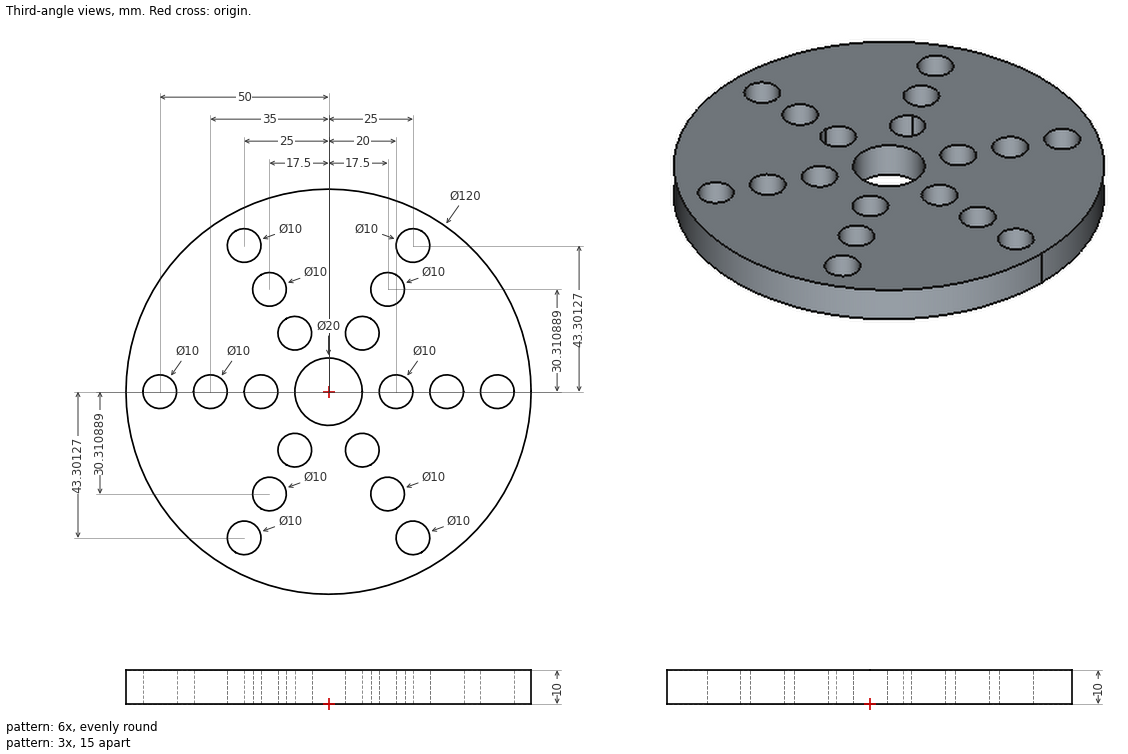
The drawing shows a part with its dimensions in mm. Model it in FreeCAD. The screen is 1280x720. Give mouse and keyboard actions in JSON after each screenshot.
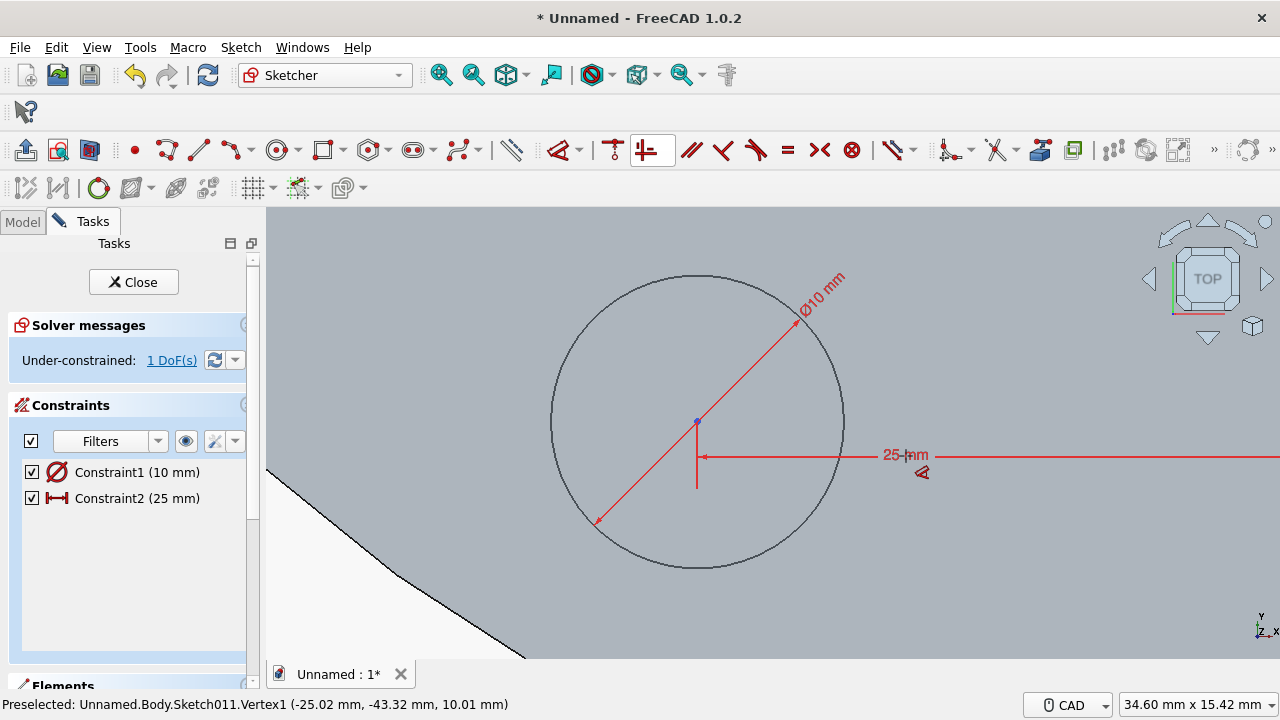
{"action": "left_click", "coordinate": [697, 422]}
{"action": "left_click", "coordinate": [663, 328]}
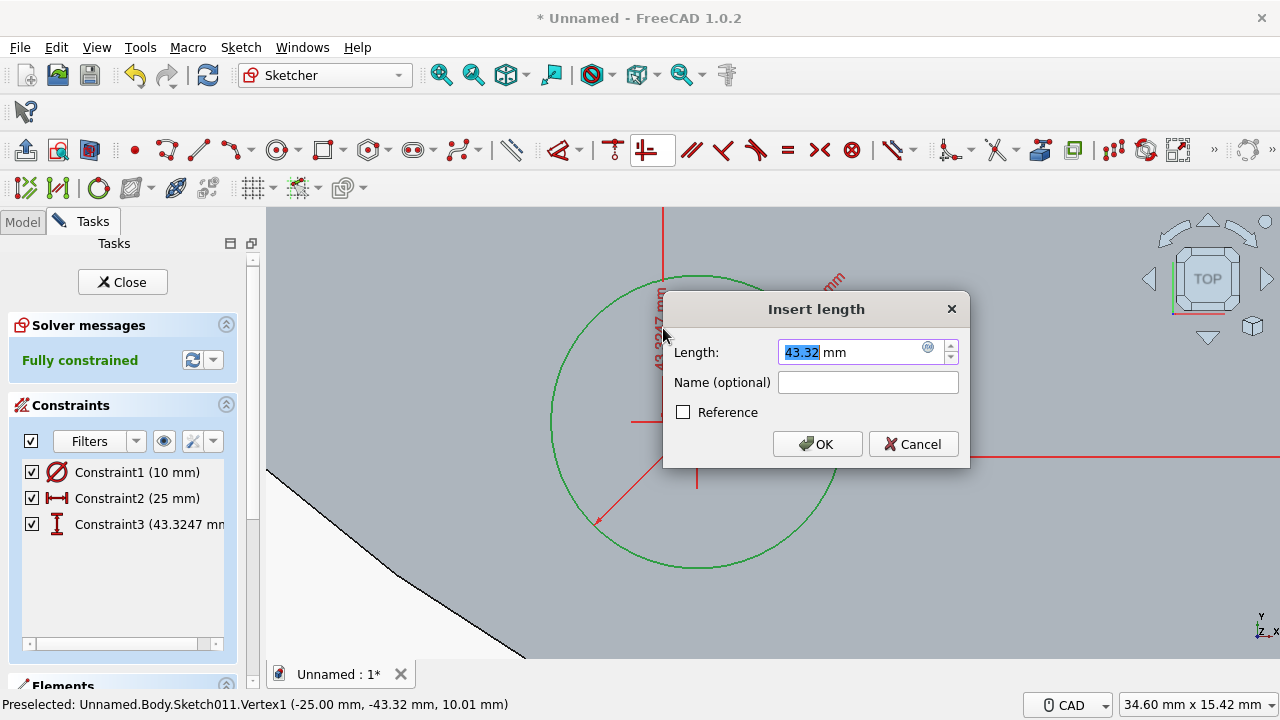
{"action": "type", "text": "43.30127"}
{"action": "key", "text": "Return"}
{"action": "key", "text": "Escape"}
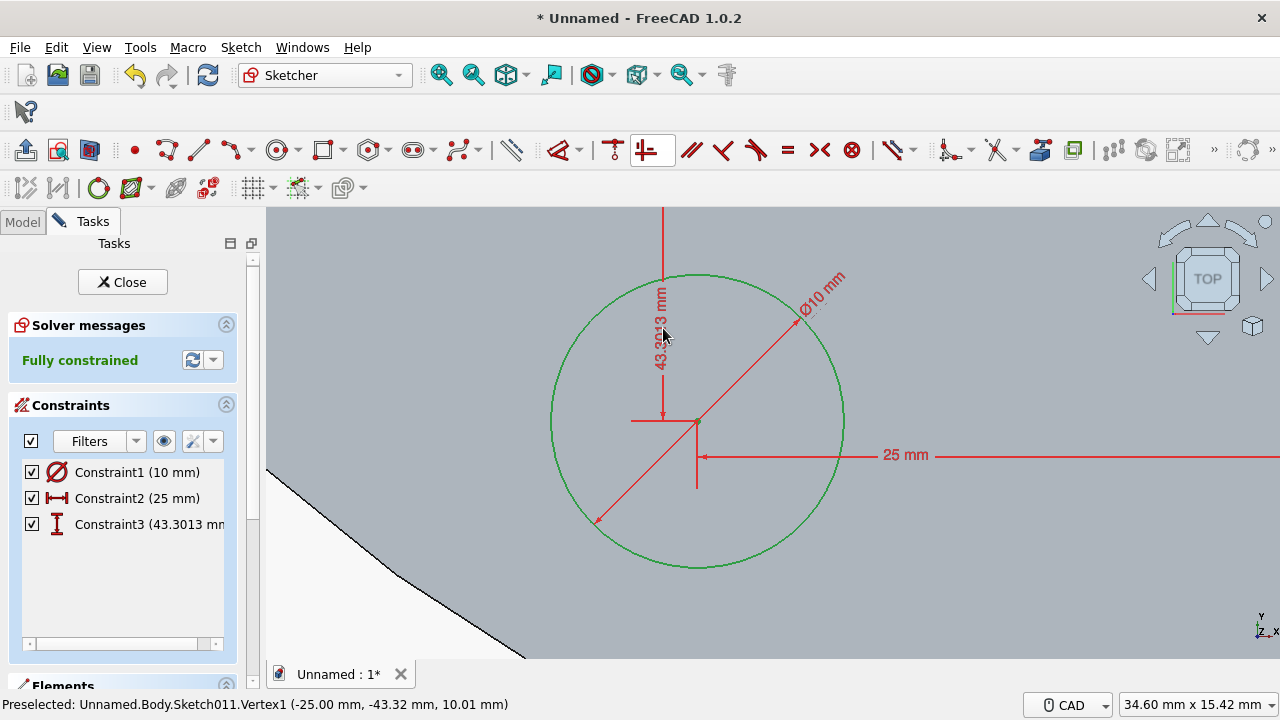
{"action": "left_click", "coordinate": [123, 282]}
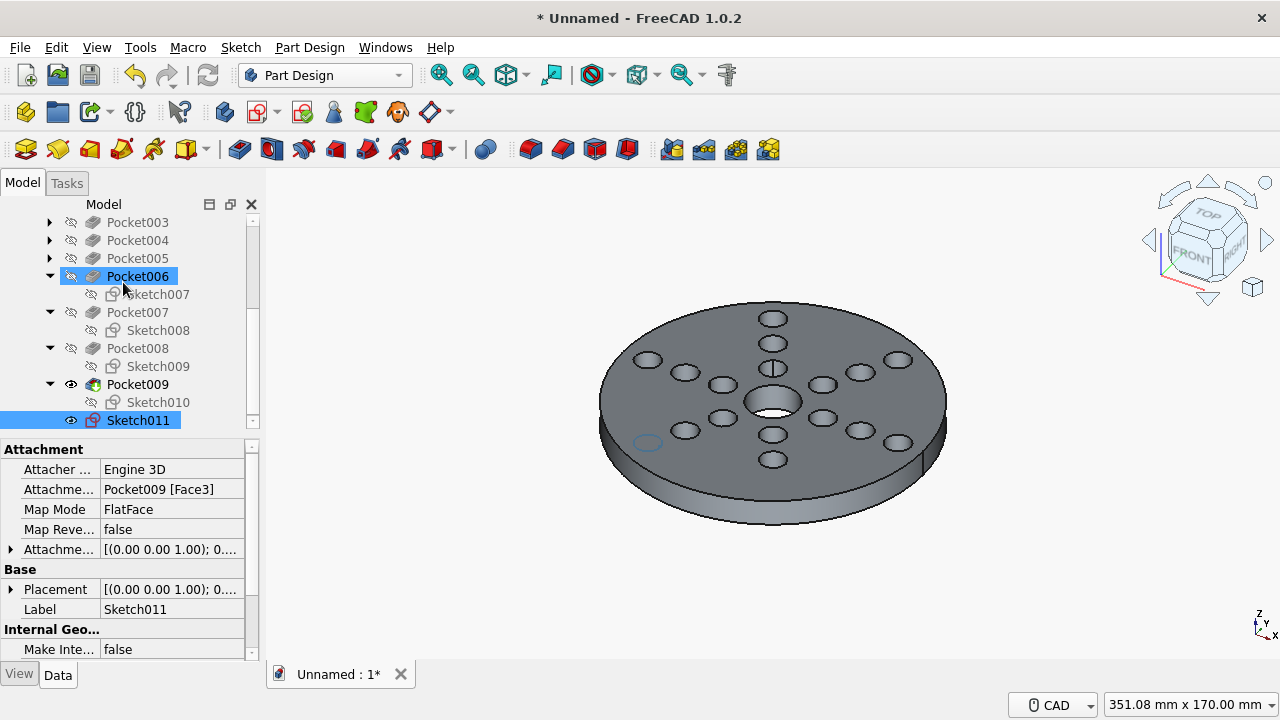
{"action": "left_click", "coordinate": [240, 150]}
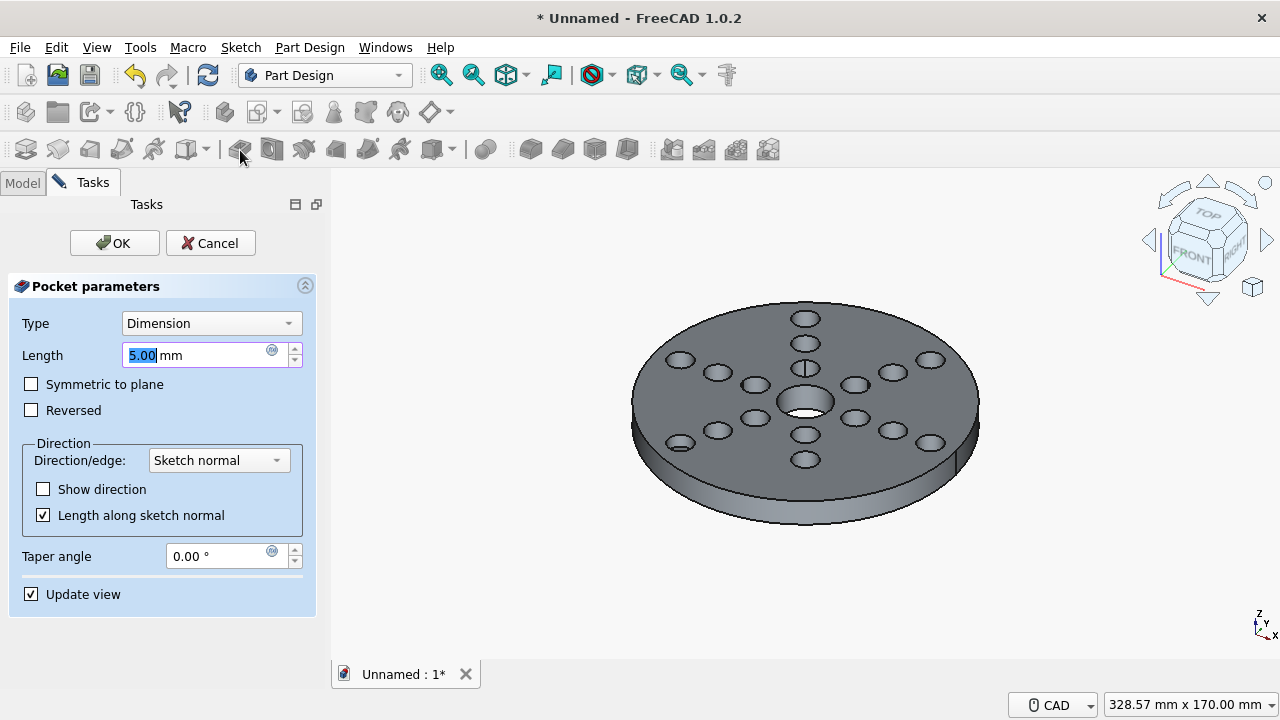
{"action": "type", "text": "10"}
{"action": "key", "text": "Tab"}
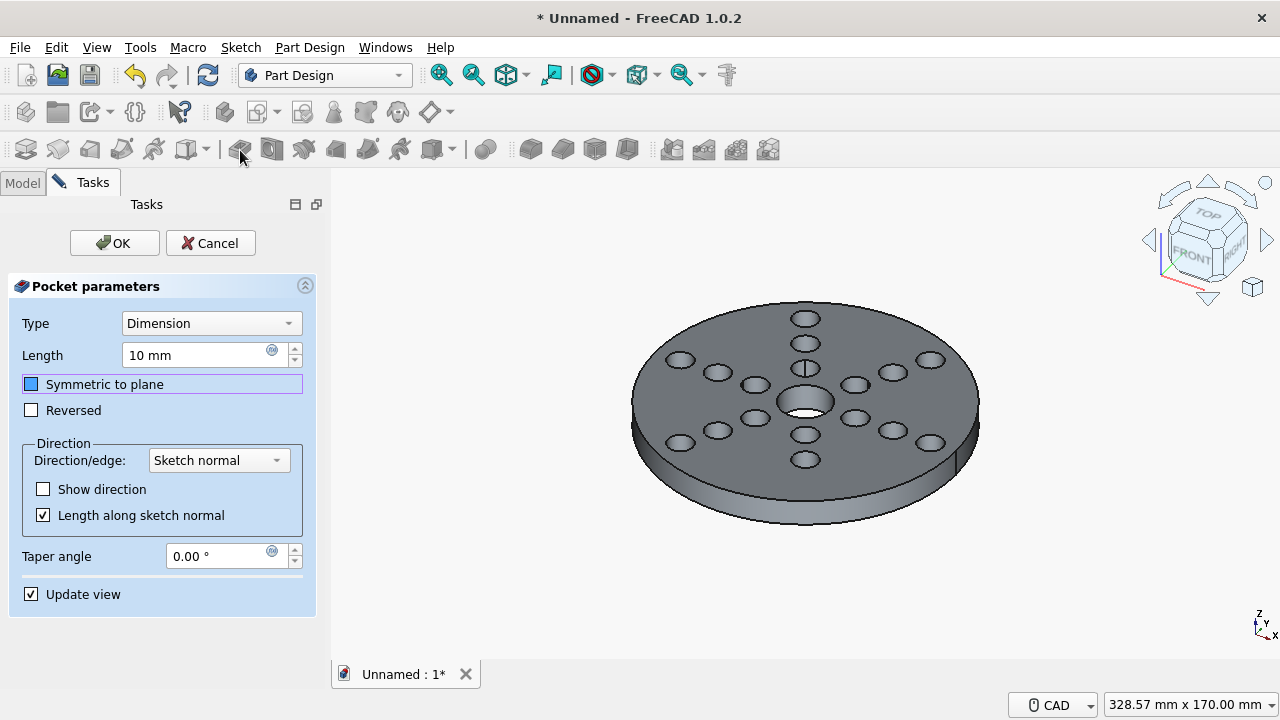
{"action": "left_click", "coordinate": [115, 243]}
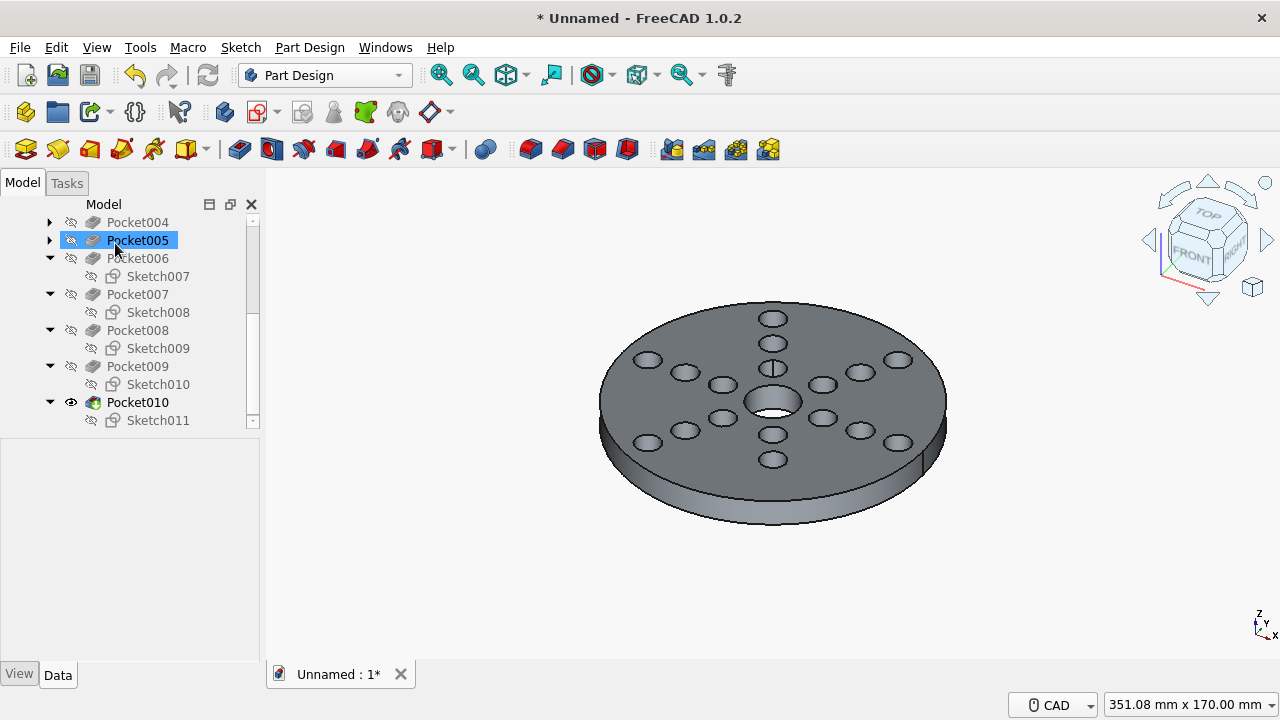
{"action": "left_click", "coordinate": [823, 351]}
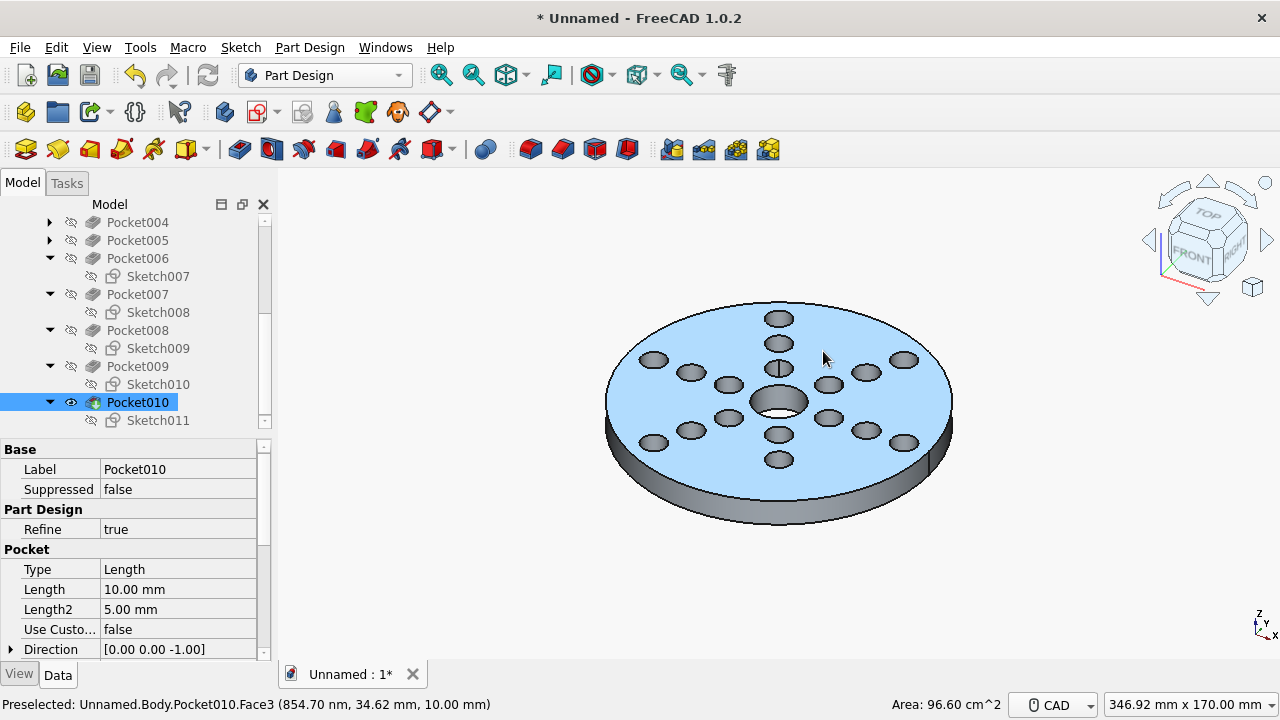
{"action": "left_click", "coordinate": [258, 112]}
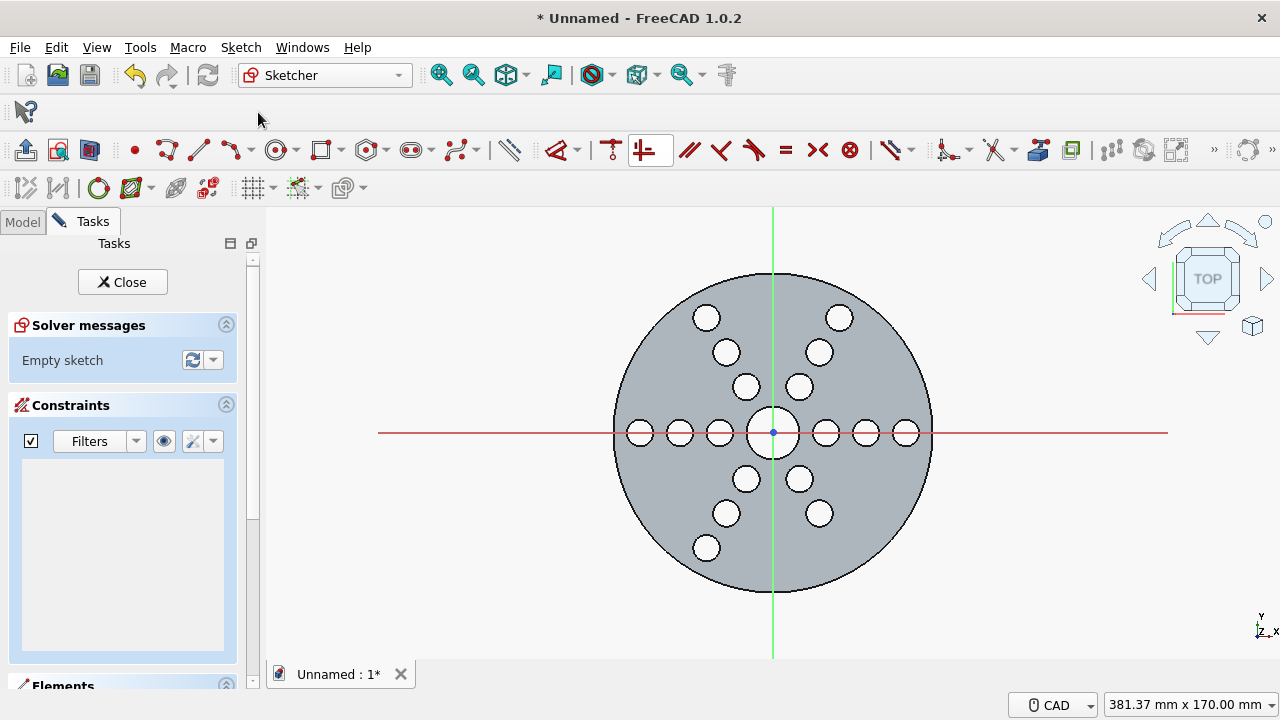
{"action": "scroll", "coordinate": [853, 560], "scroll_direction": "up", "scroll_amount": 12}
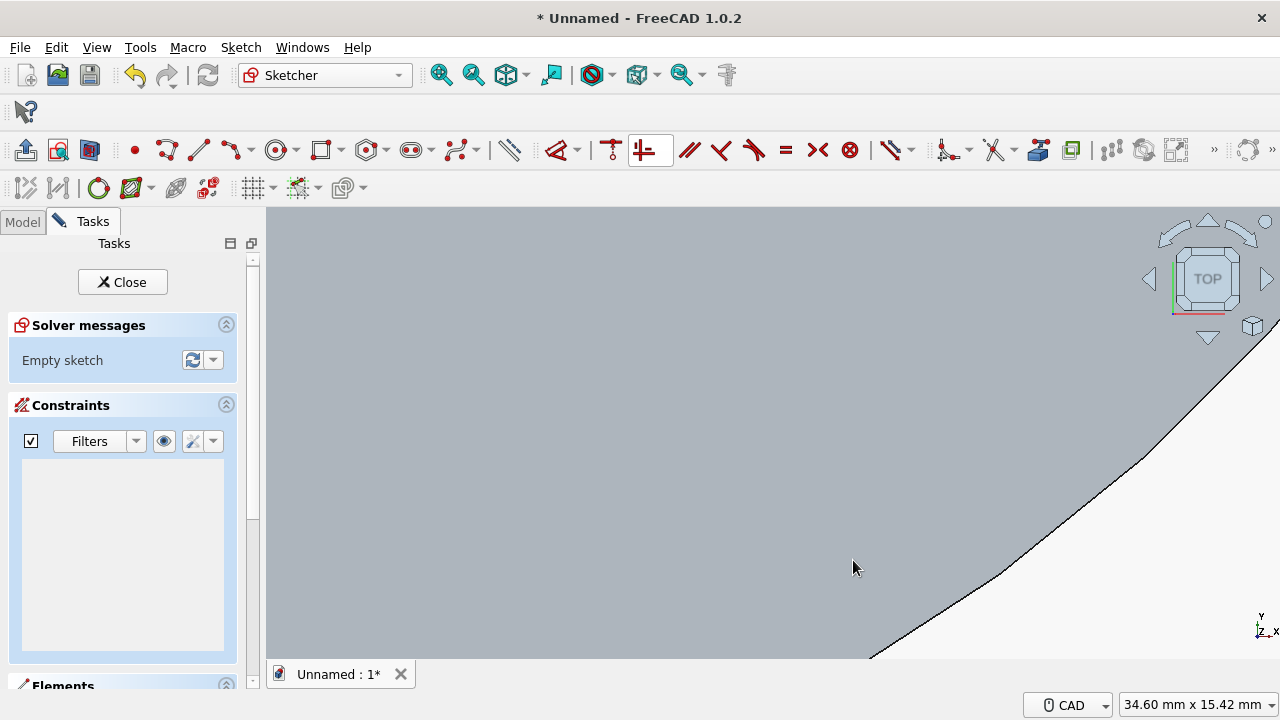
{"action": "left_click", "coordinate": [276, 150]}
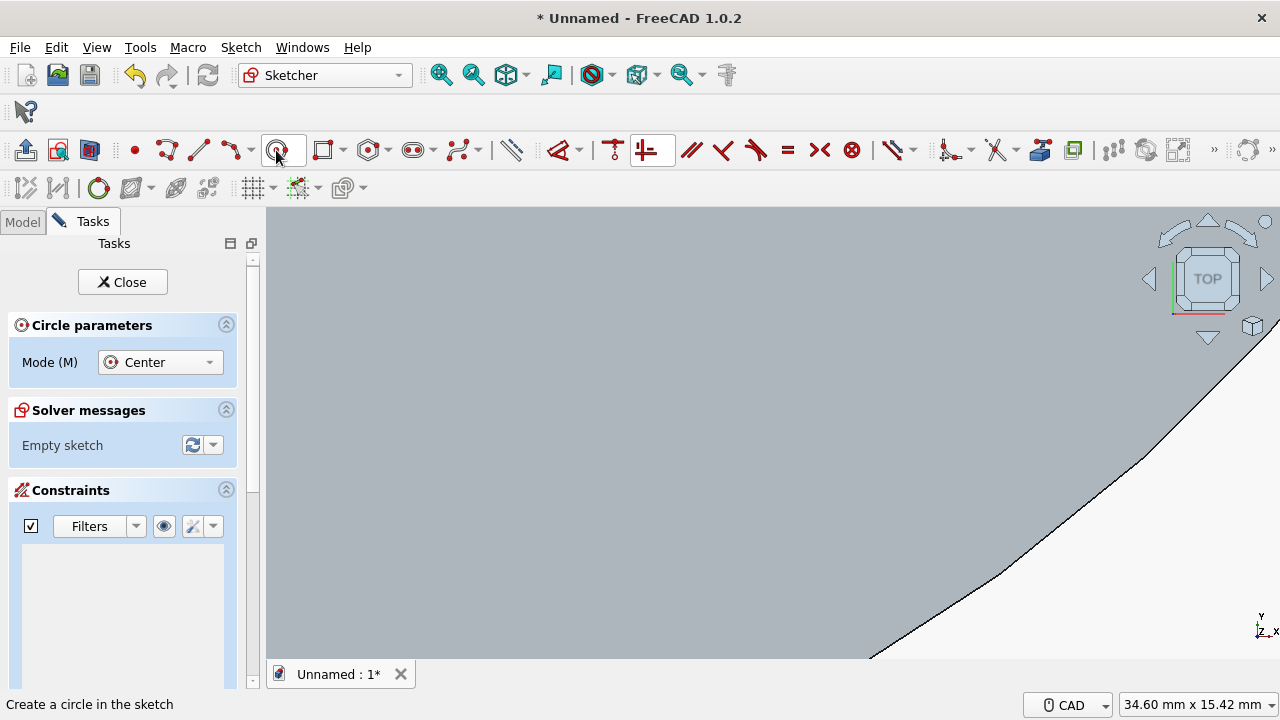
{"action": "left_click", "coordinate": [698, 421]}
{"action": "left_click", "coordinate": [802, 318]}
{"action": "key", "text": "Escape"}